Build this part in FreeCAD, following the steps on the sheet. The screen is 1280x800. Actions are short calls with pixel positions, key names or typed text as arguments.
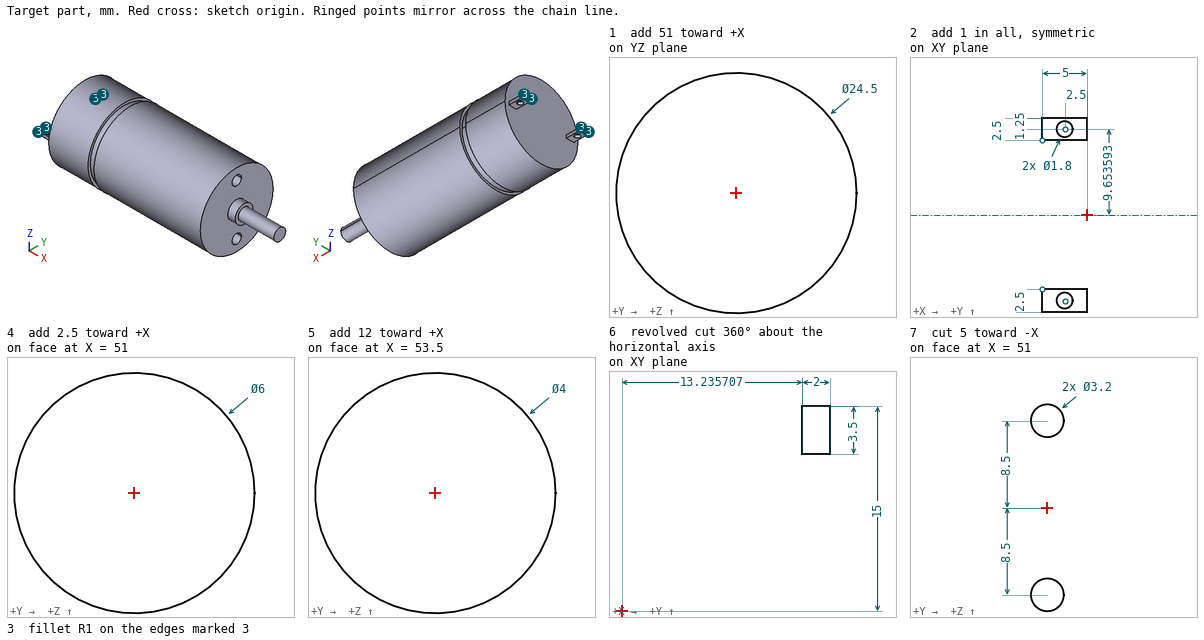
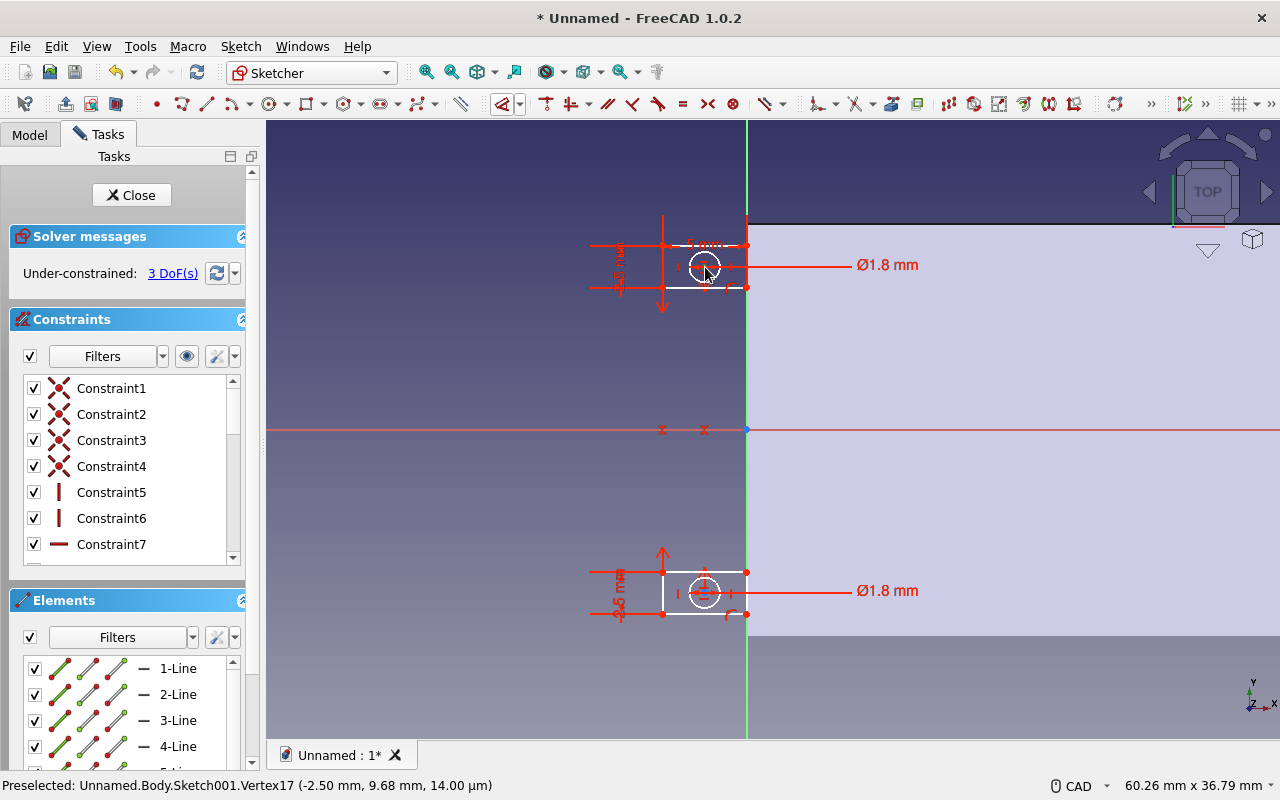
click(520, 104)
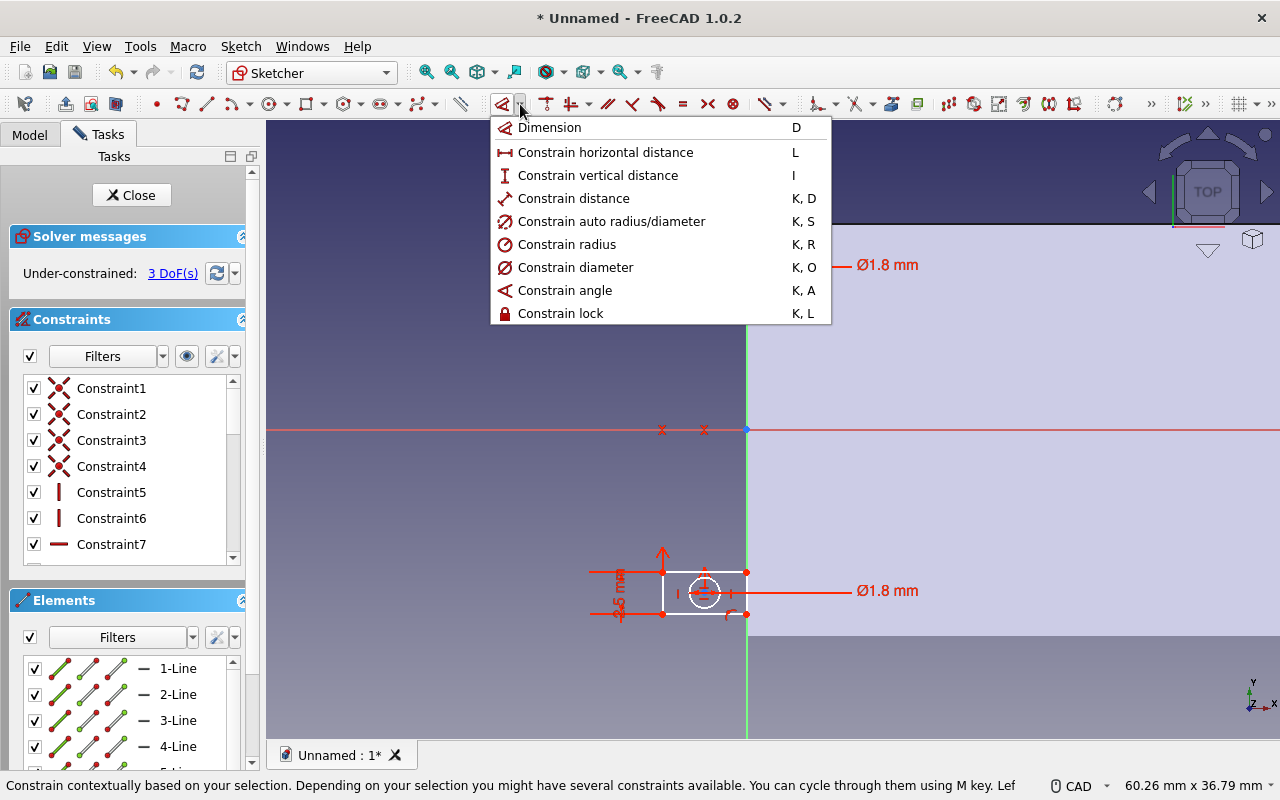
click(661, 152)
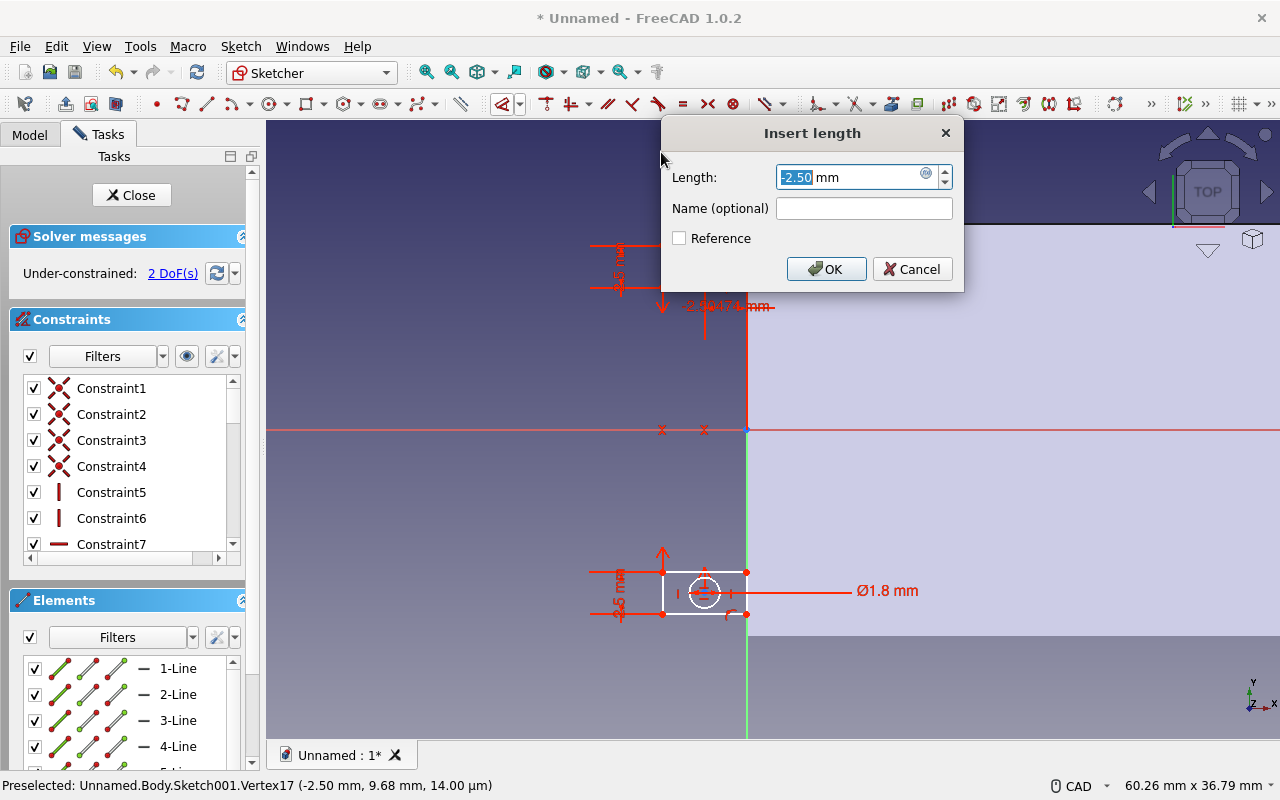
text(-2.5)
key(Return)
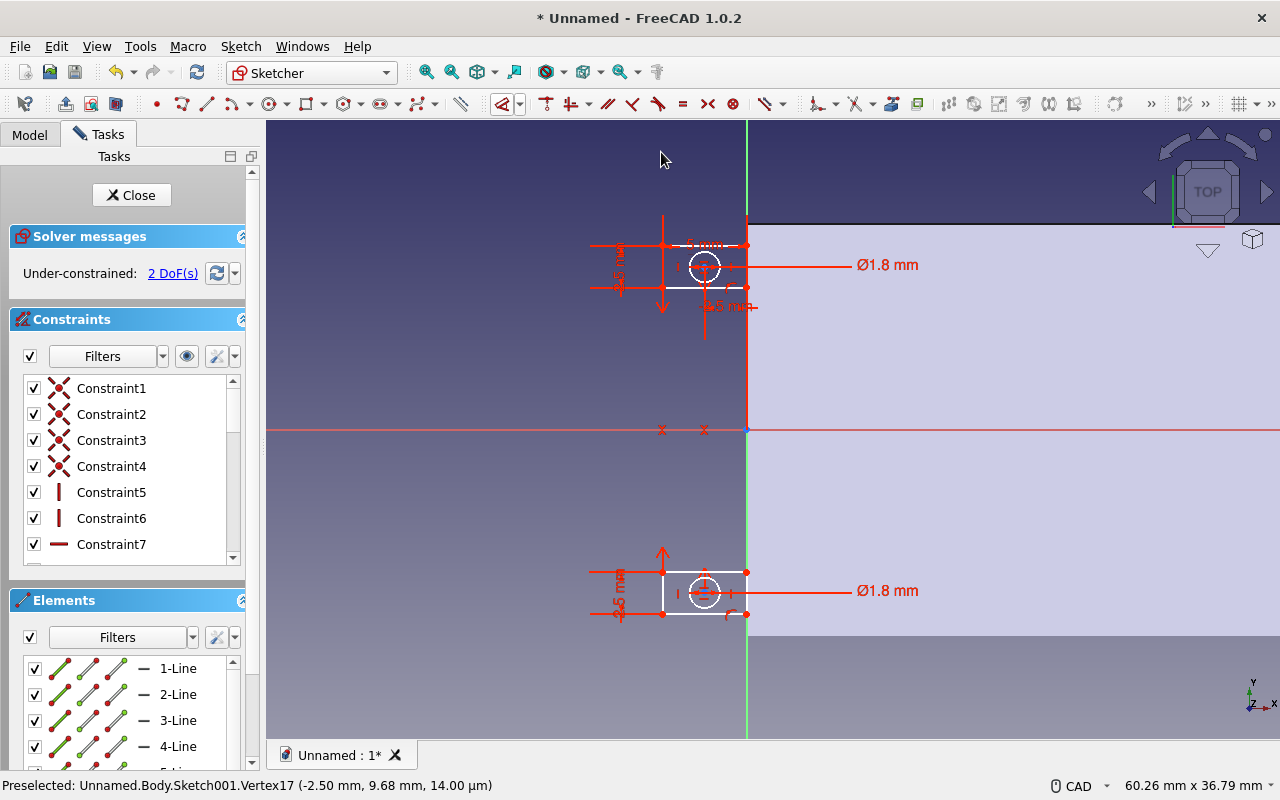
scroll(663, 246, up, 4)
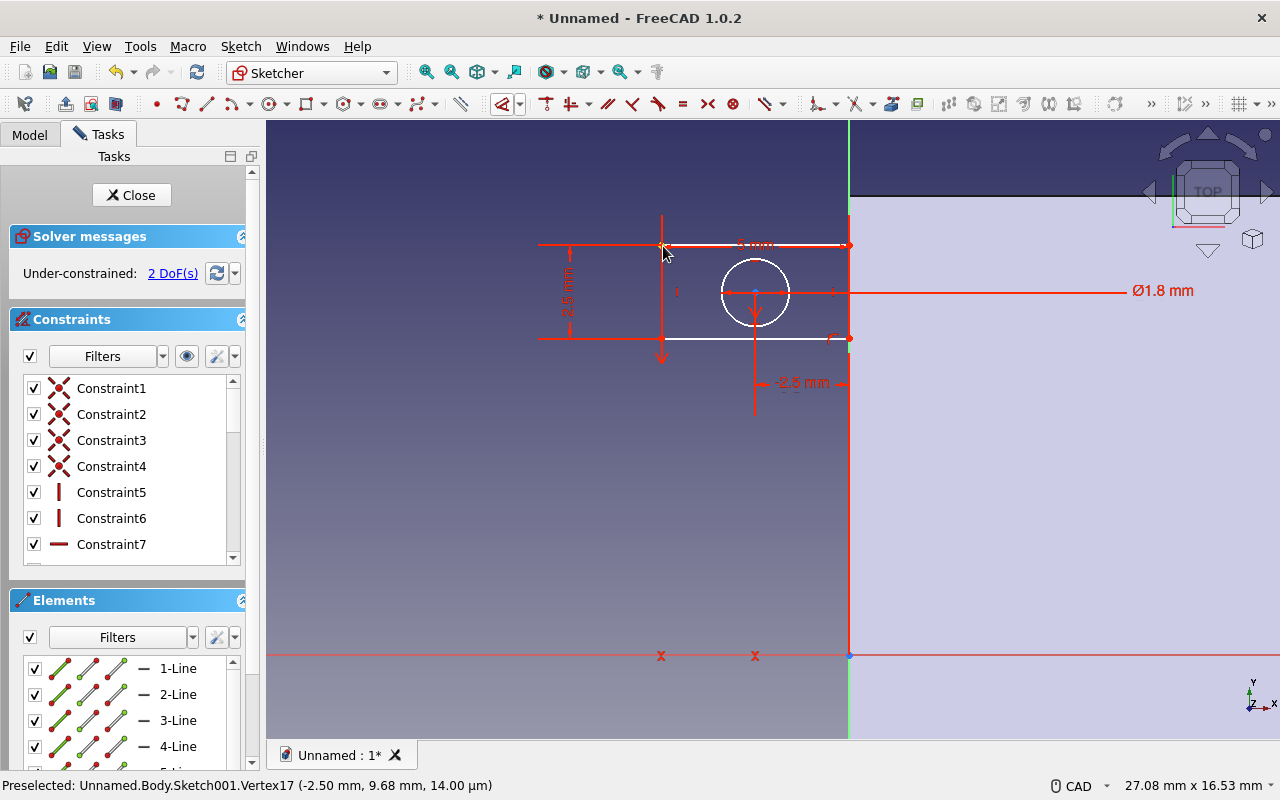
click(662, 245)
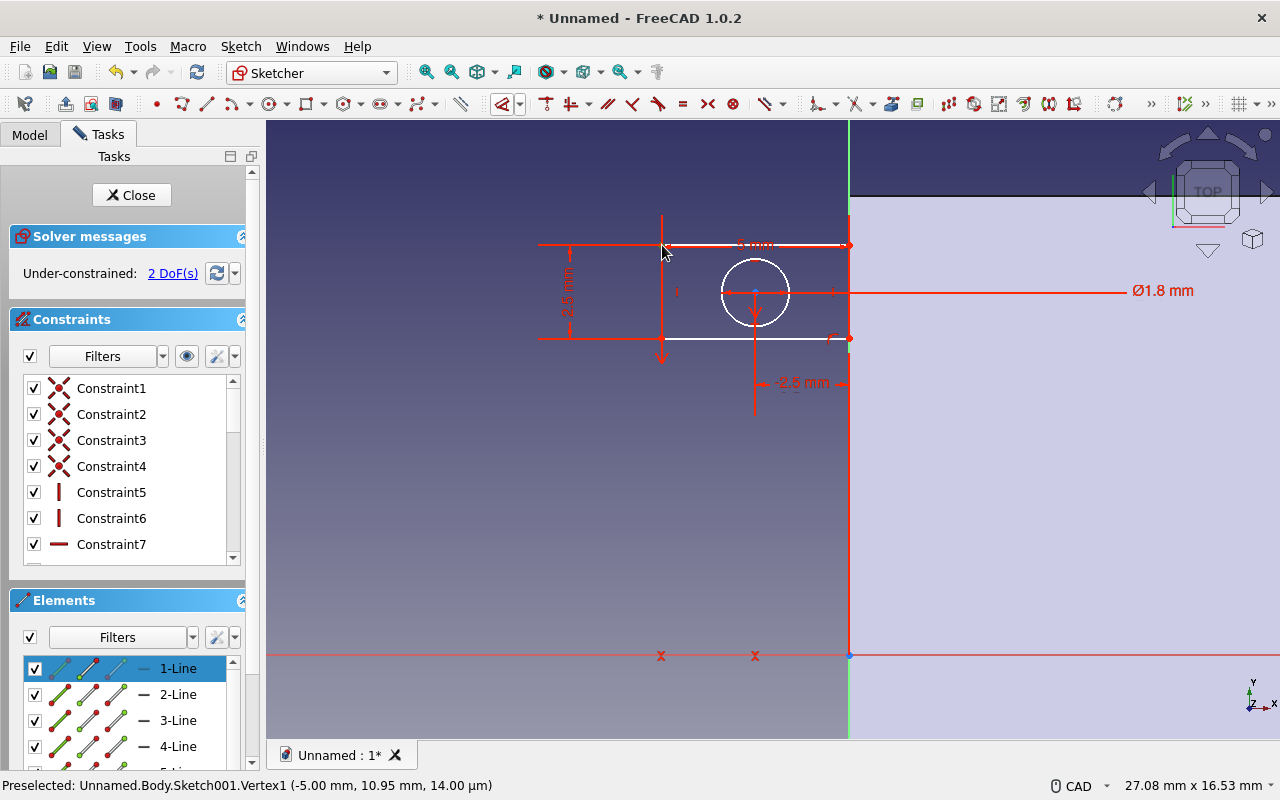
click(755, 293)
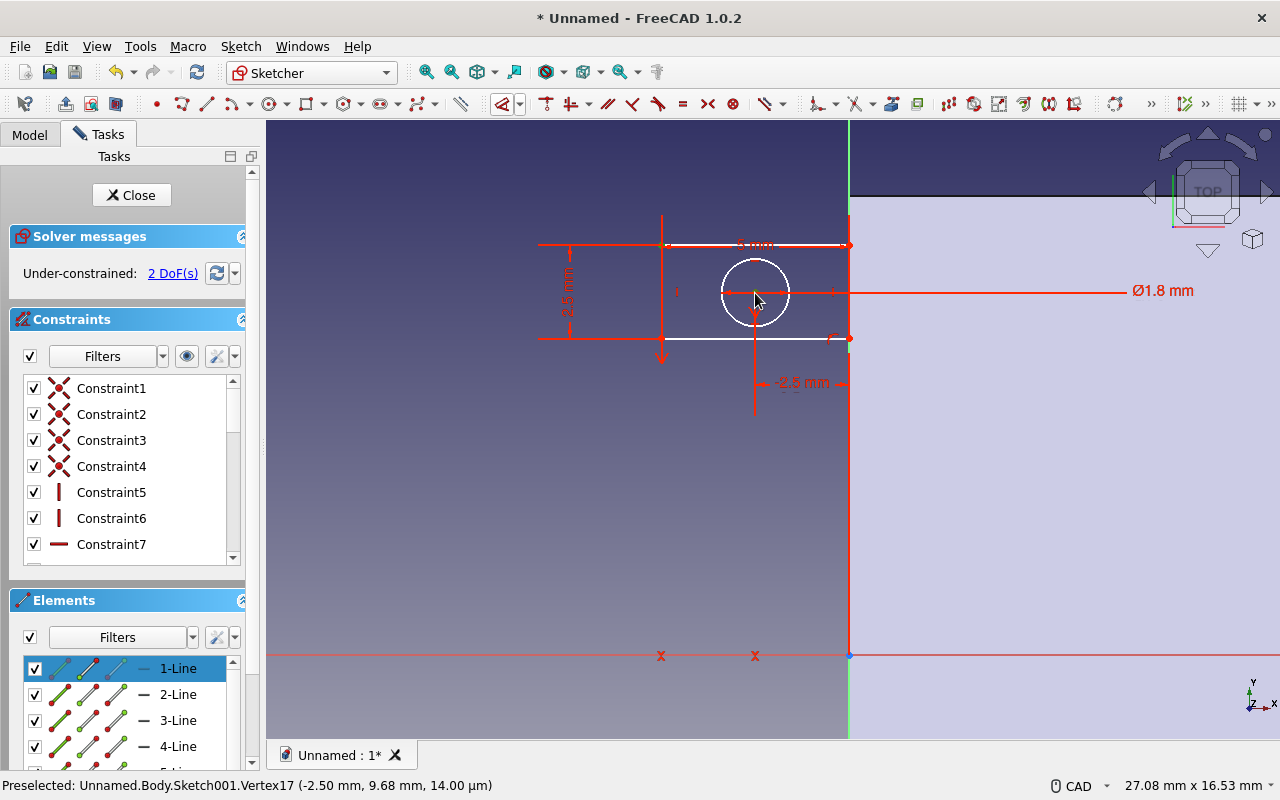
click(520, 104)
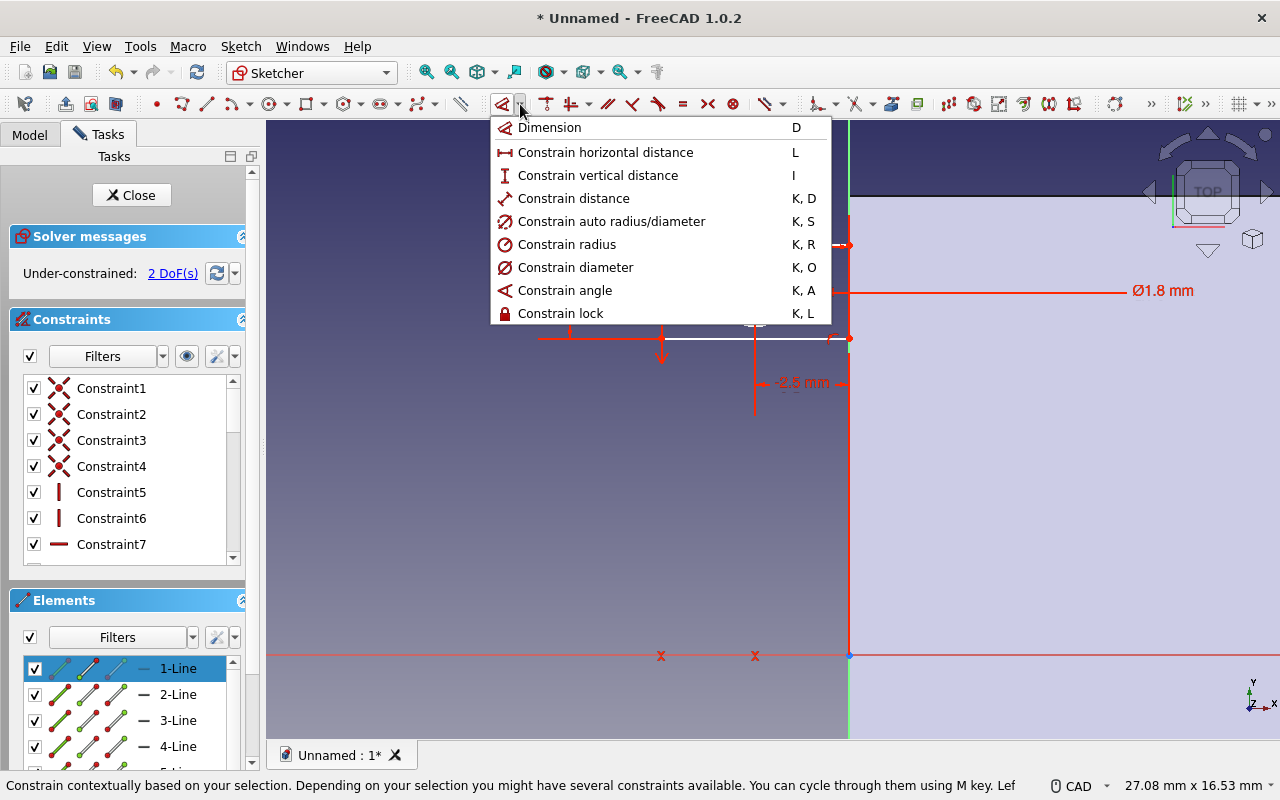
click(661, 176)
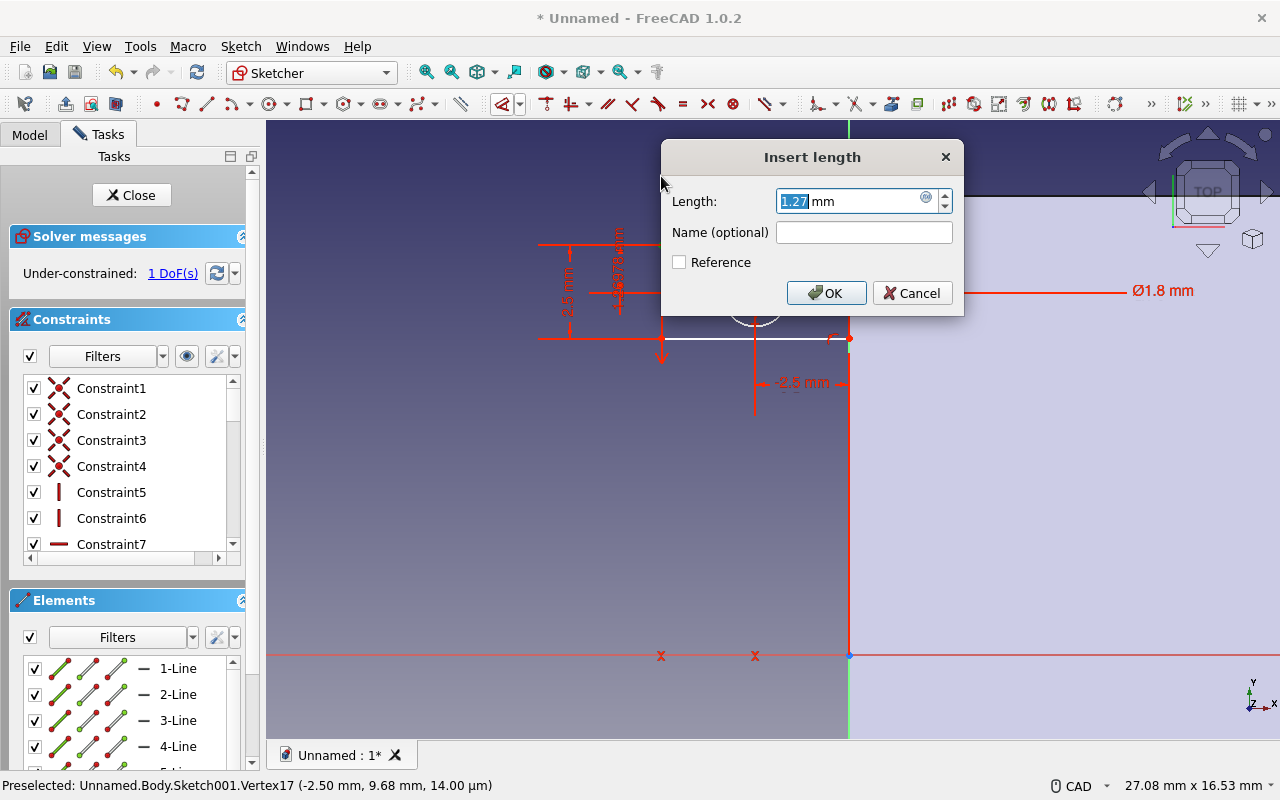
text(1.25)
key(Return)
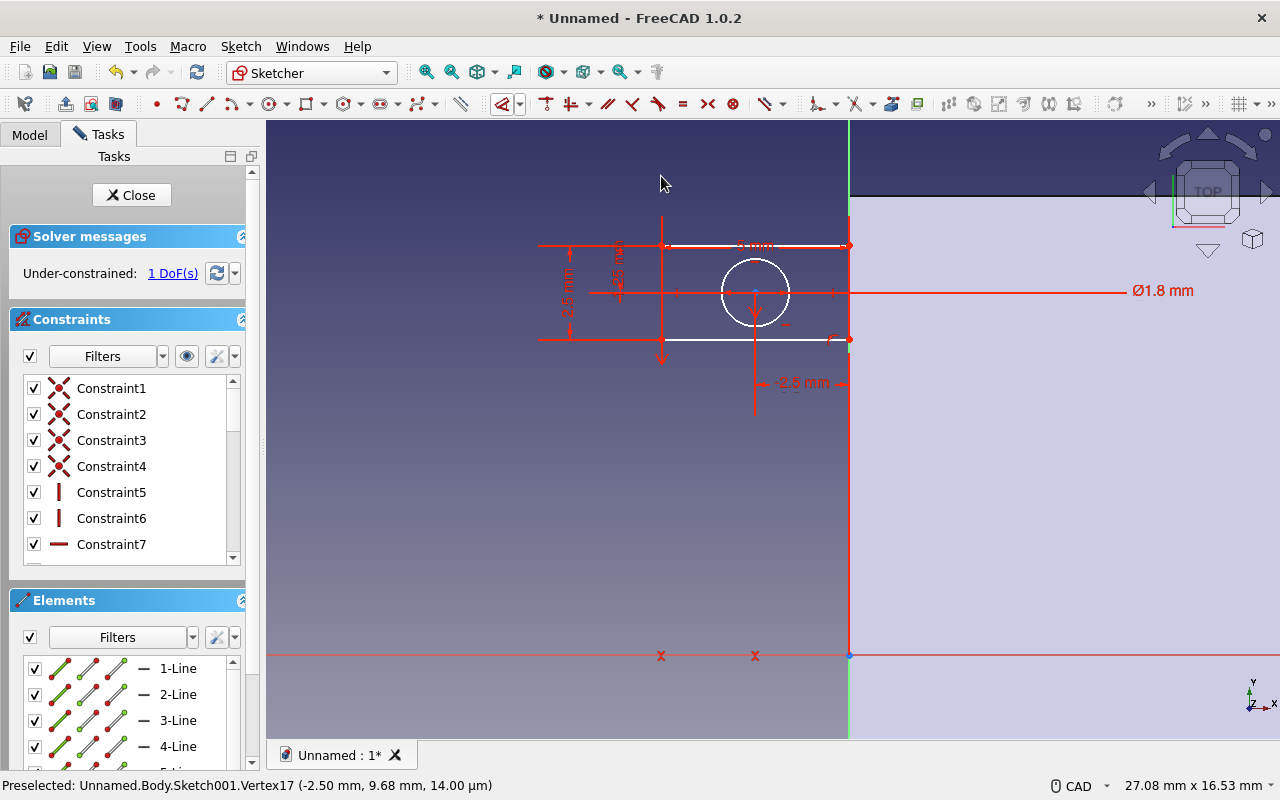
click(755, 293)